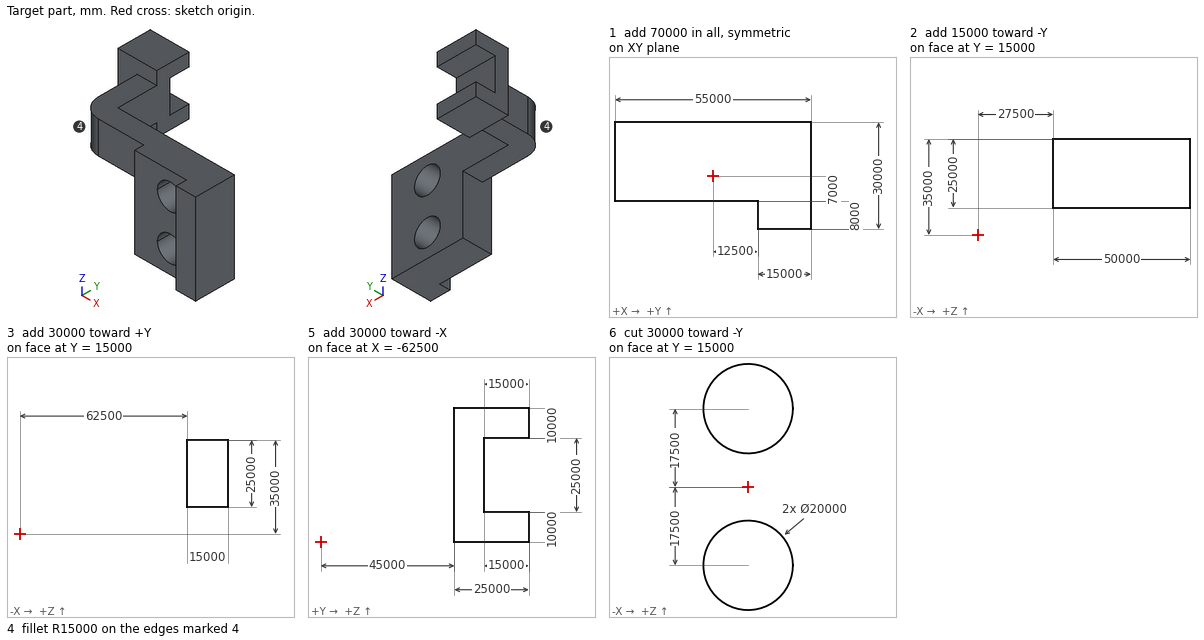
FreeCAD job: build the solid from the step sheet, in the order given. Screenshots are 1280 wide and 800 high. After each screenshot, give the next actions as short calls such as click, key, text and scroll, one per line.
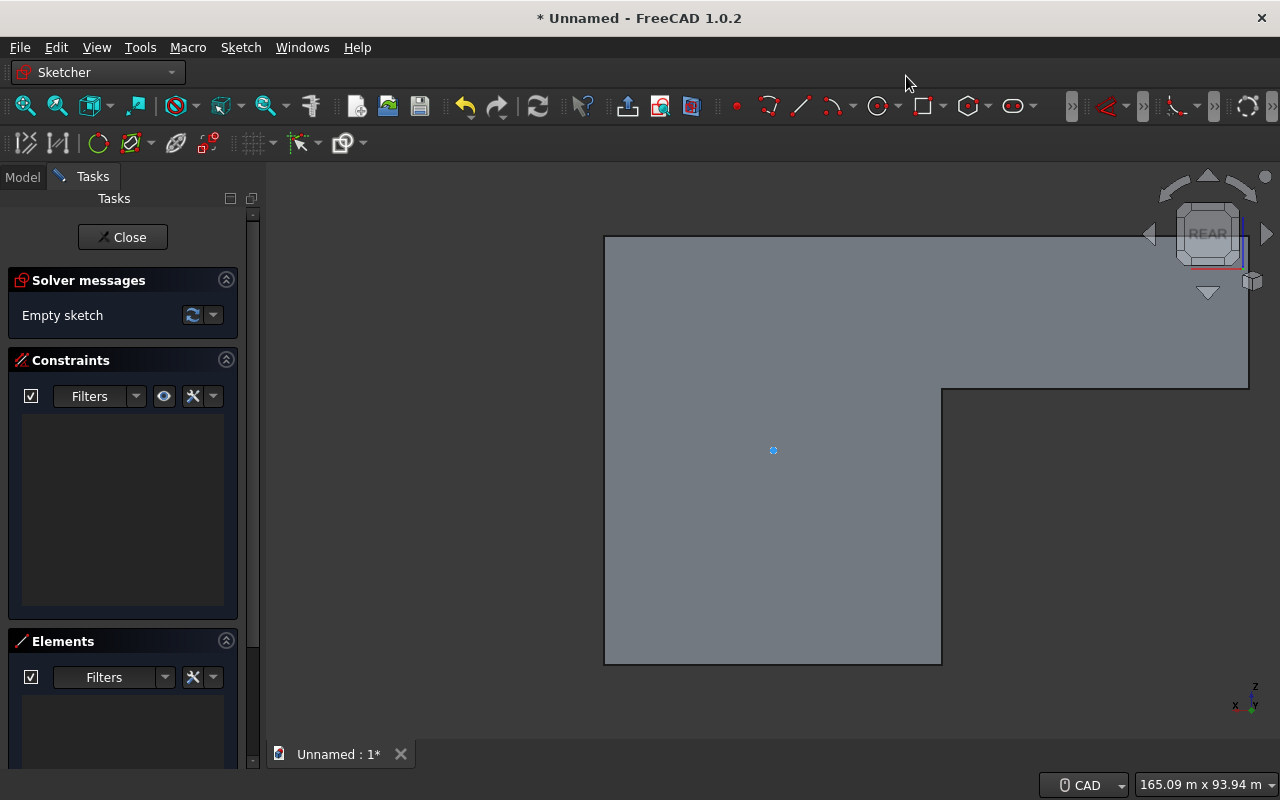
scroll(704, 450, down, 5)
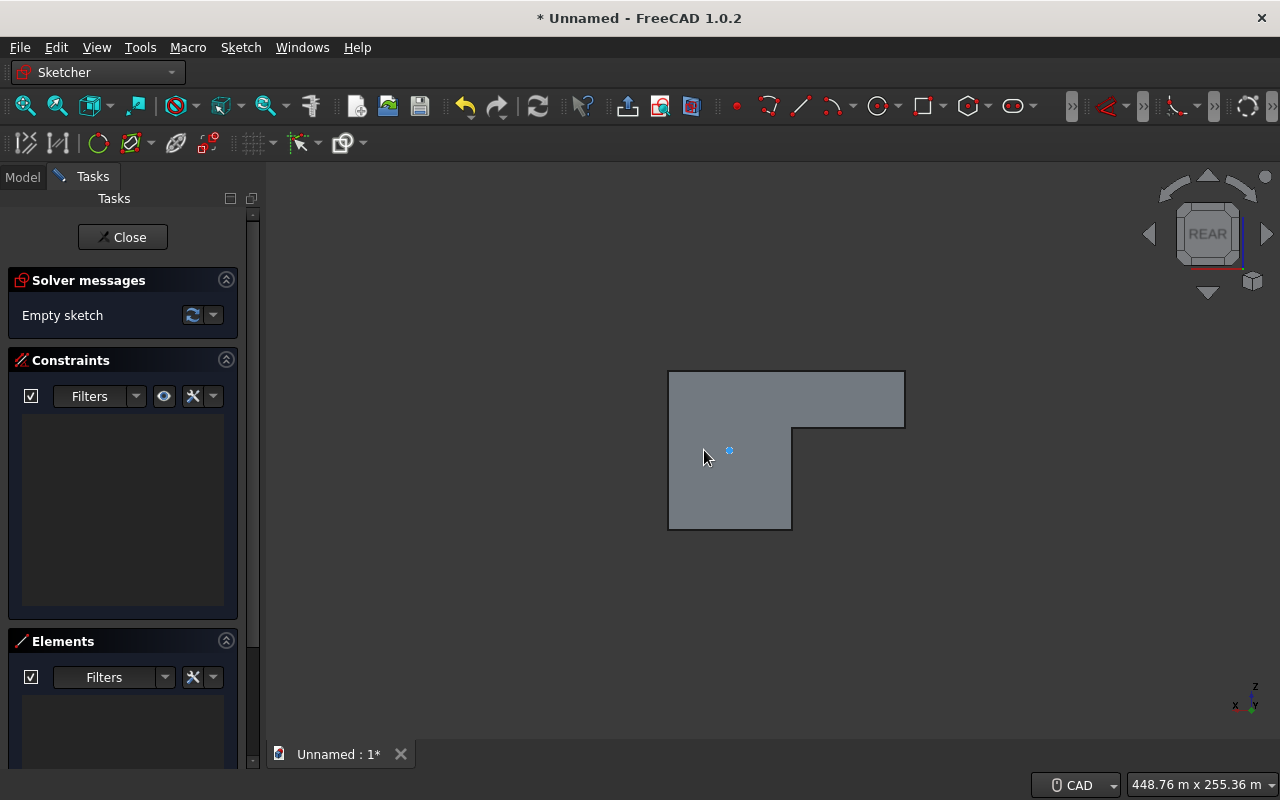
scroll(924, 390, up, 9)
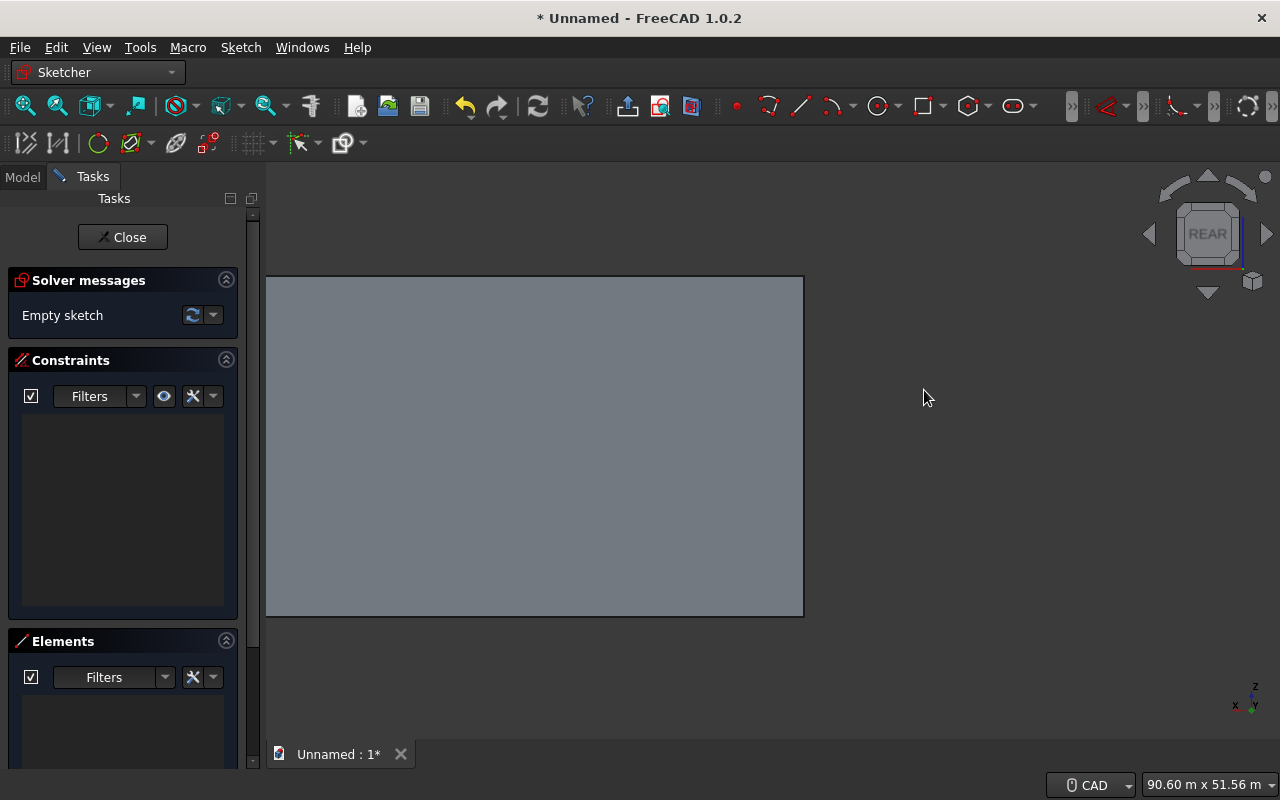
key(g)
key(r)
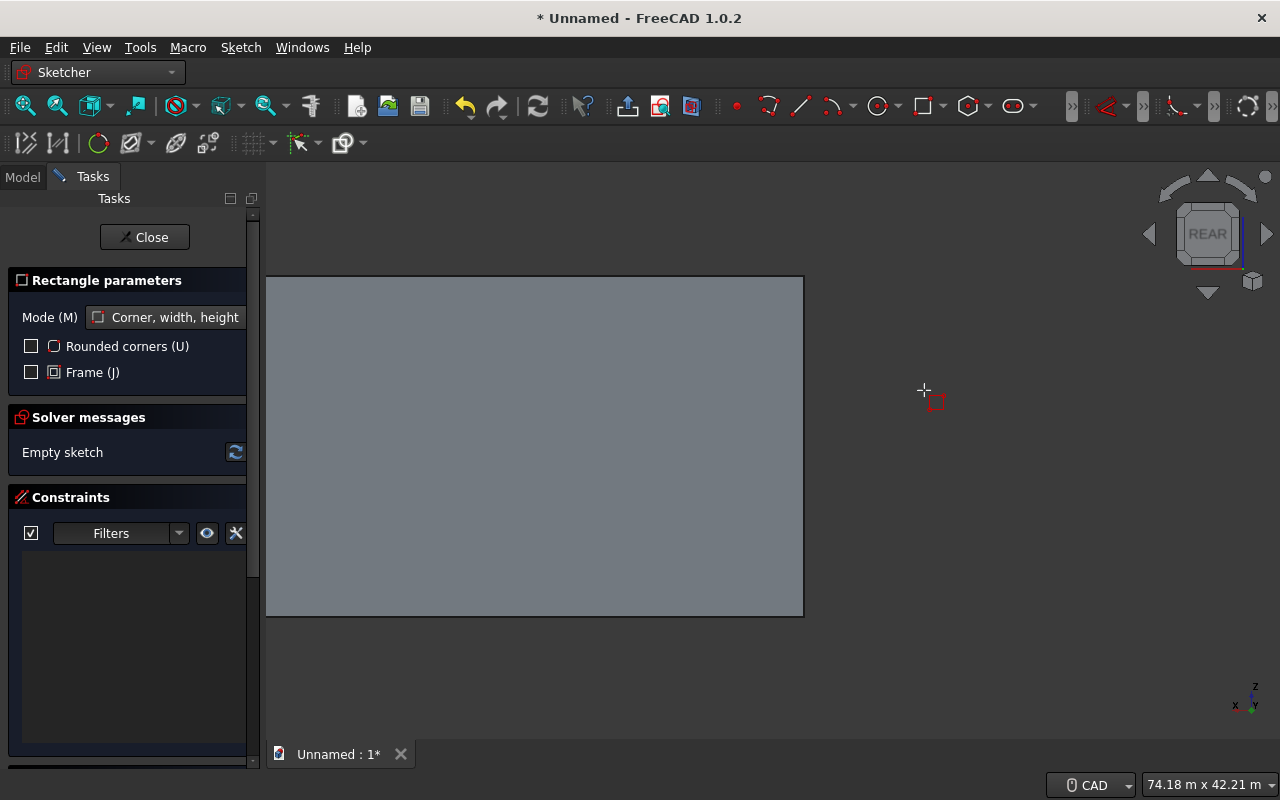
click(599, 276)
click(804, 617)
key(Escape)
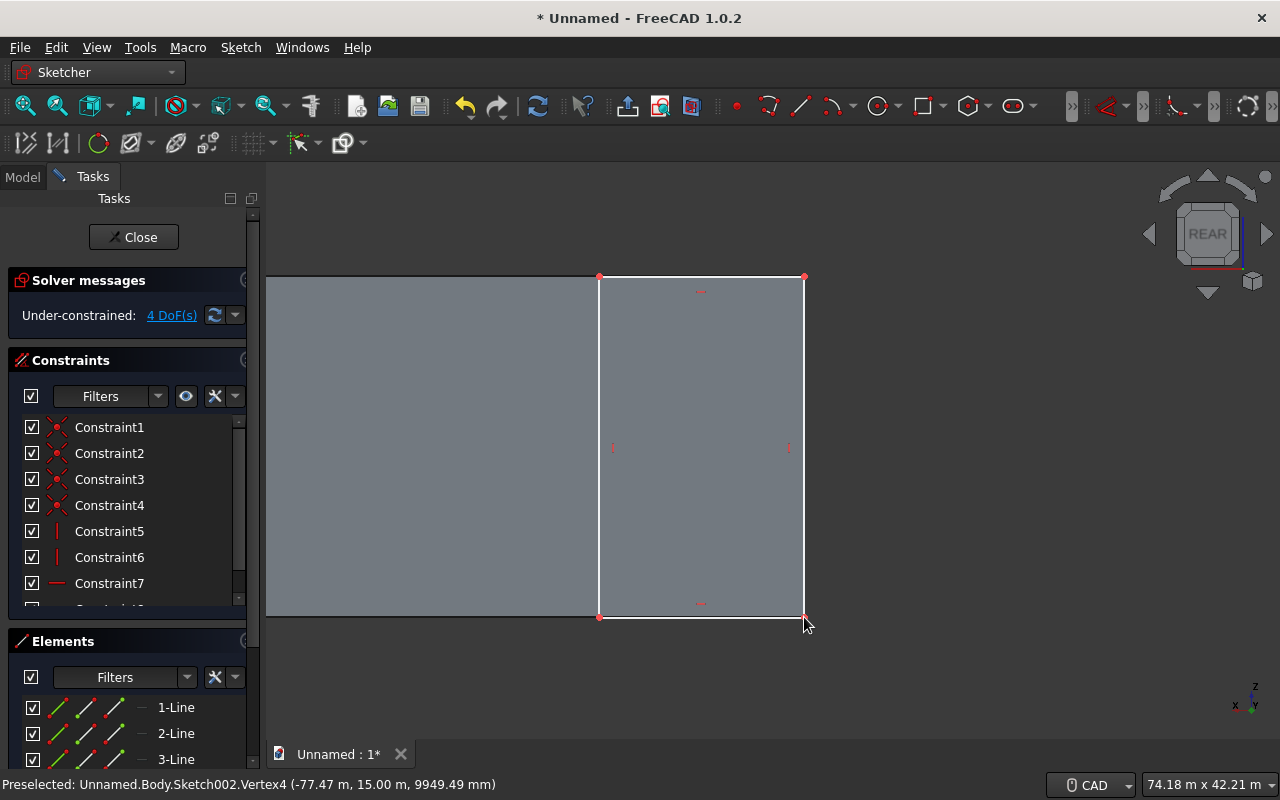
key(d)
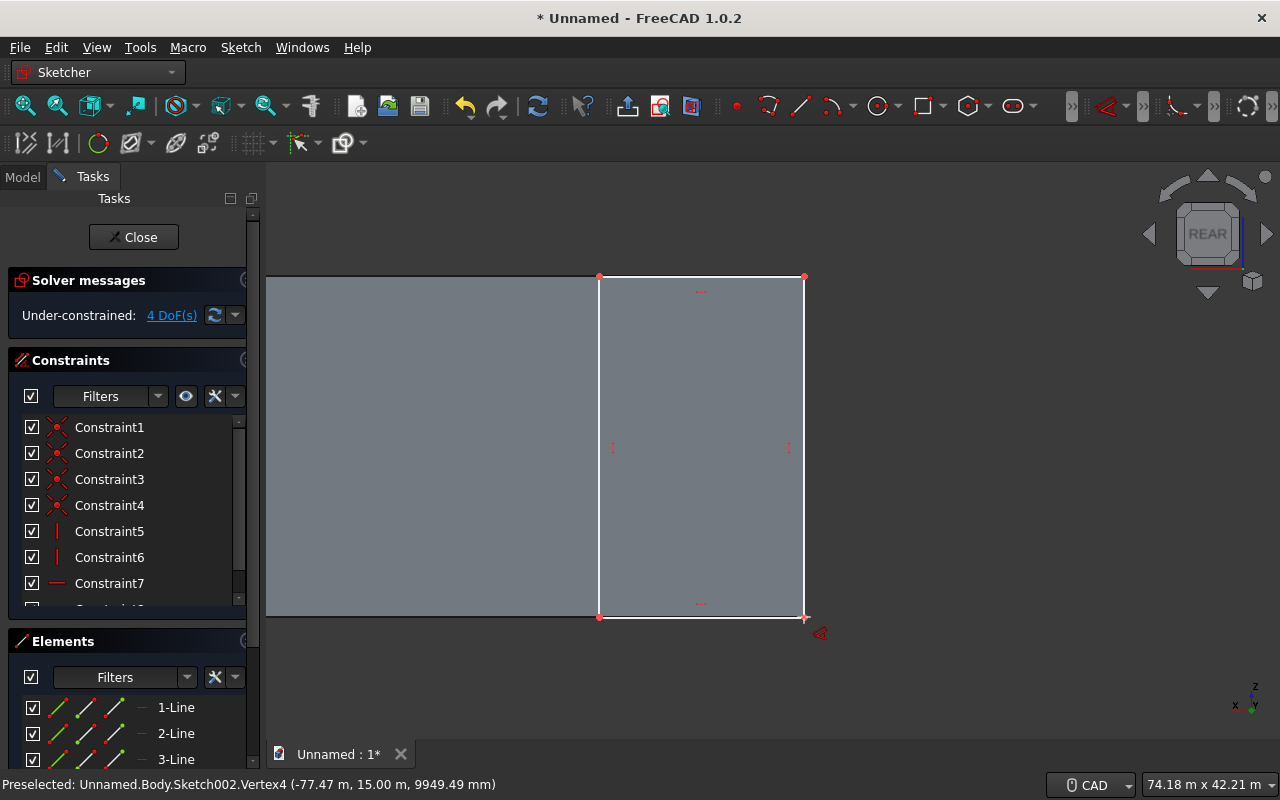
click(599, 379)
click(565, 448)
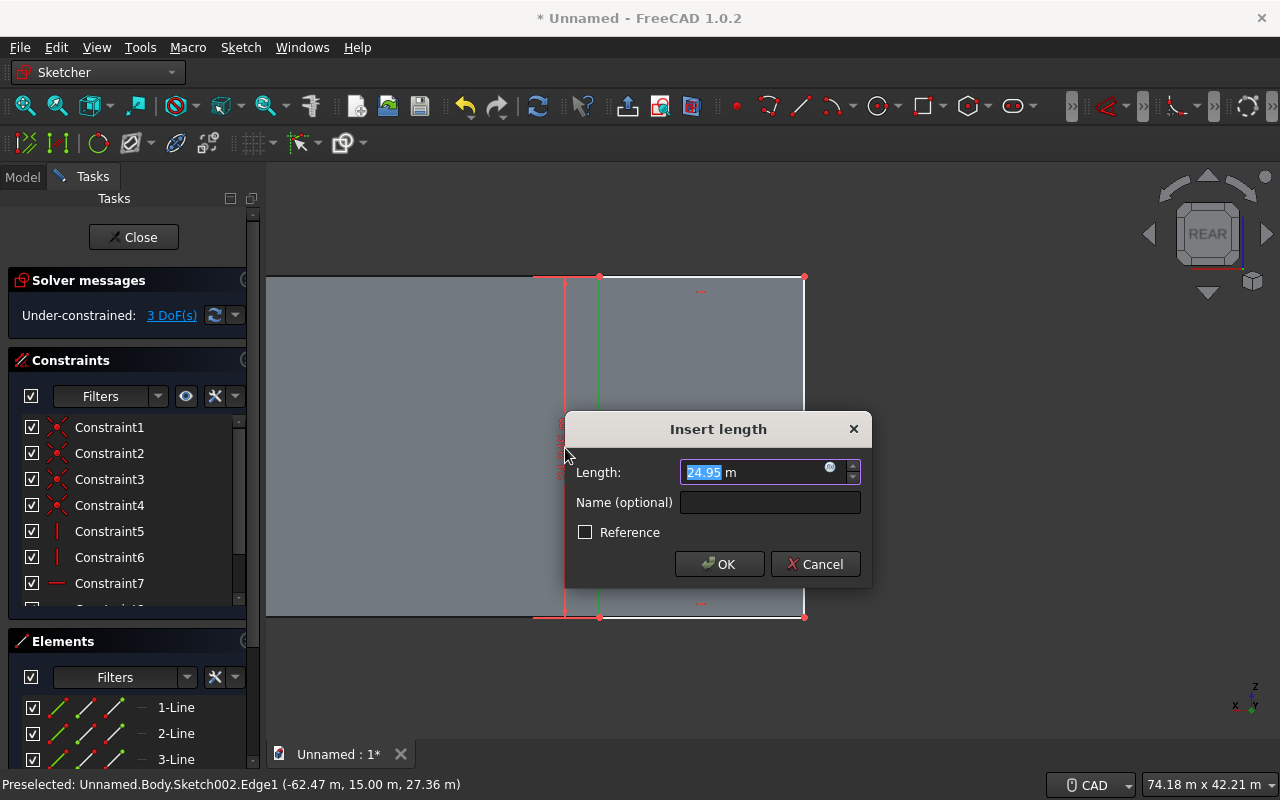
key(ctrl+a)
text(25000 mm)
key(Return)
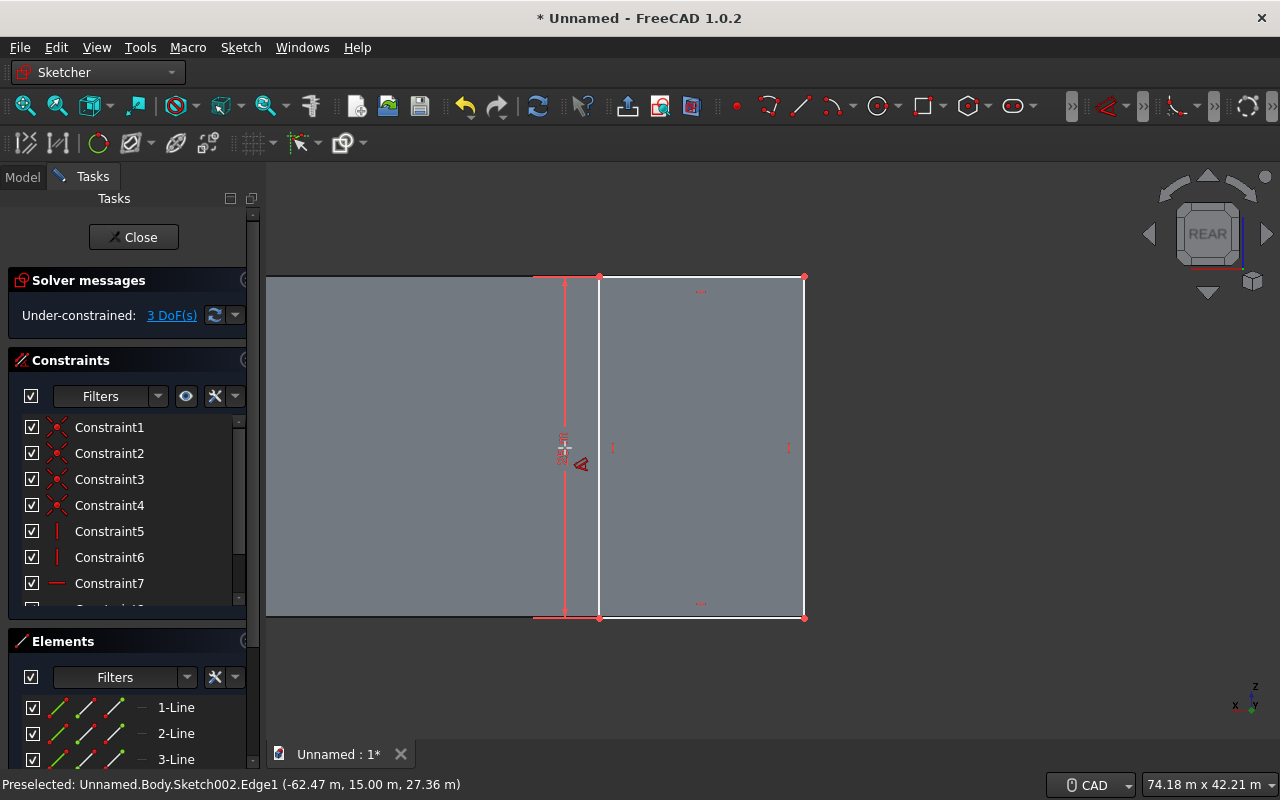
click(661, 618)
click(702, 652)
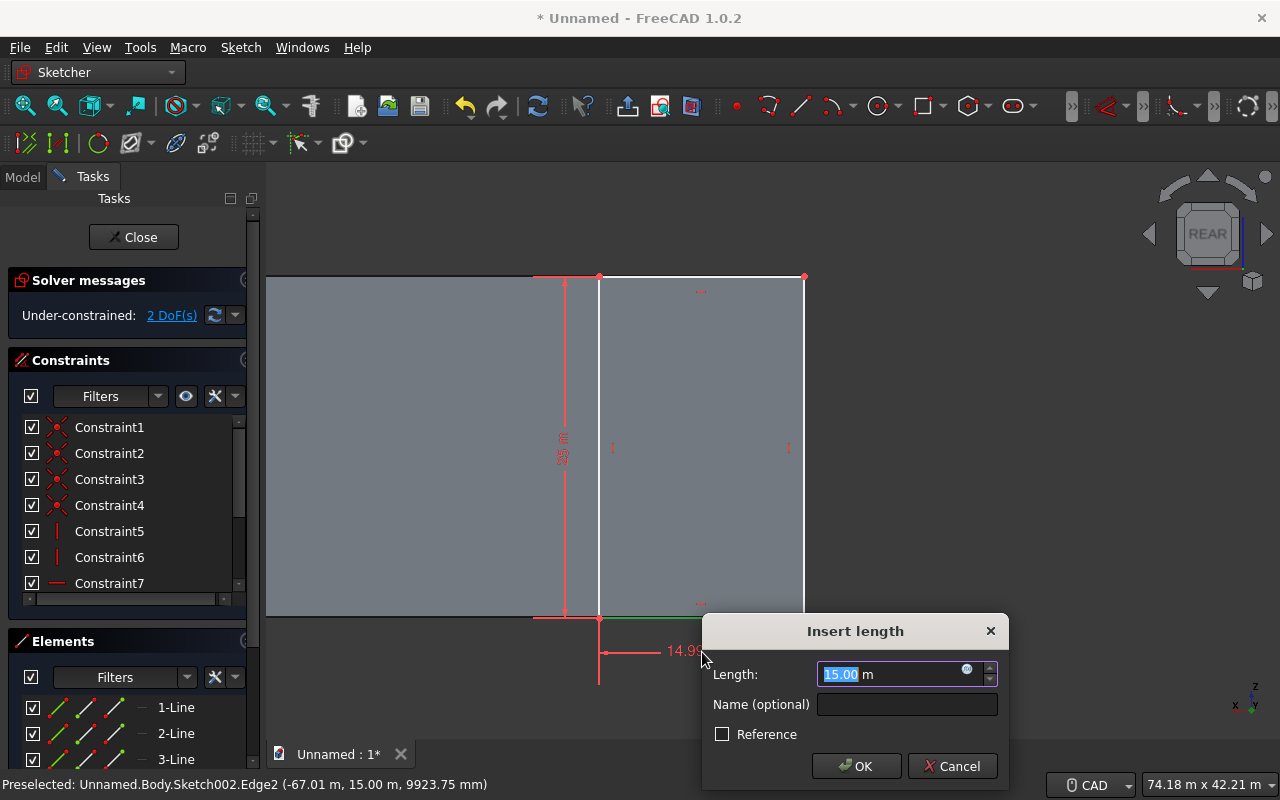
key(ctrl+a)
text(15000 mm)
key(Return)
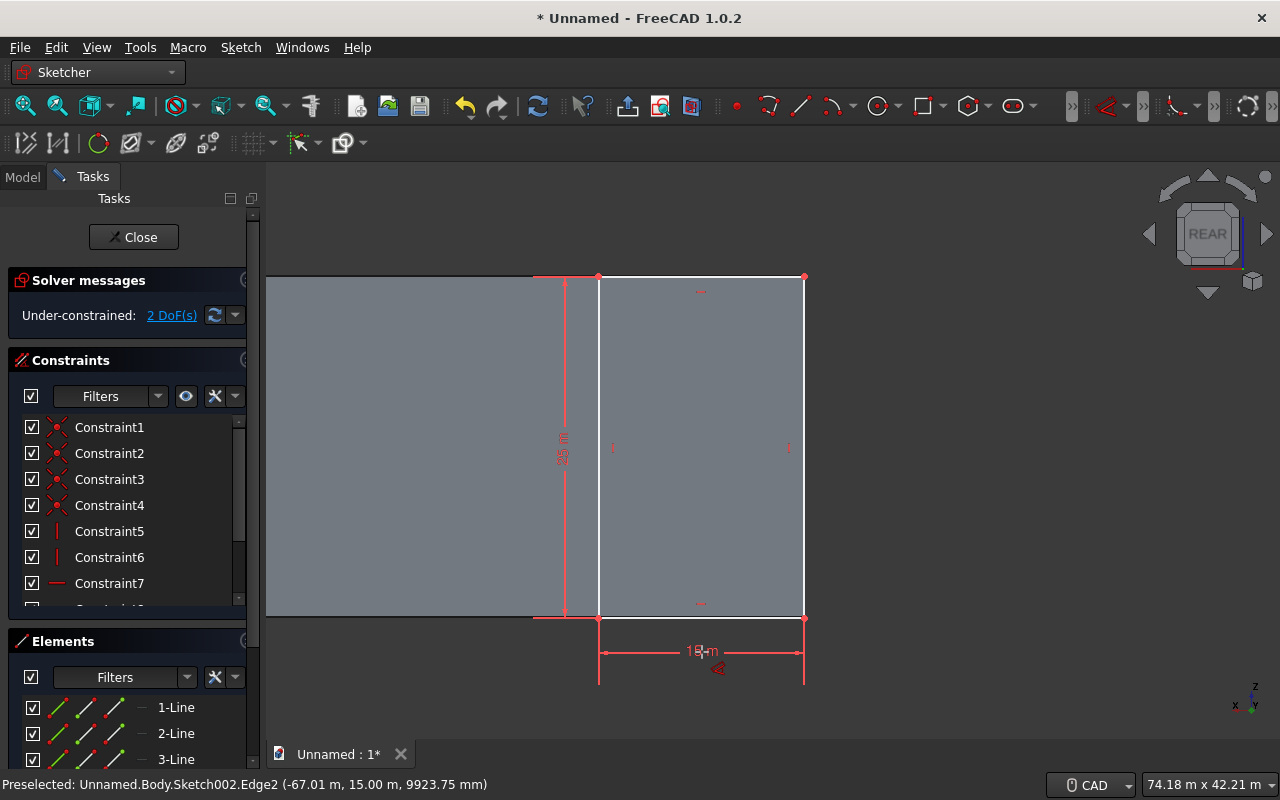
click(599, 277)
click(446, 243)